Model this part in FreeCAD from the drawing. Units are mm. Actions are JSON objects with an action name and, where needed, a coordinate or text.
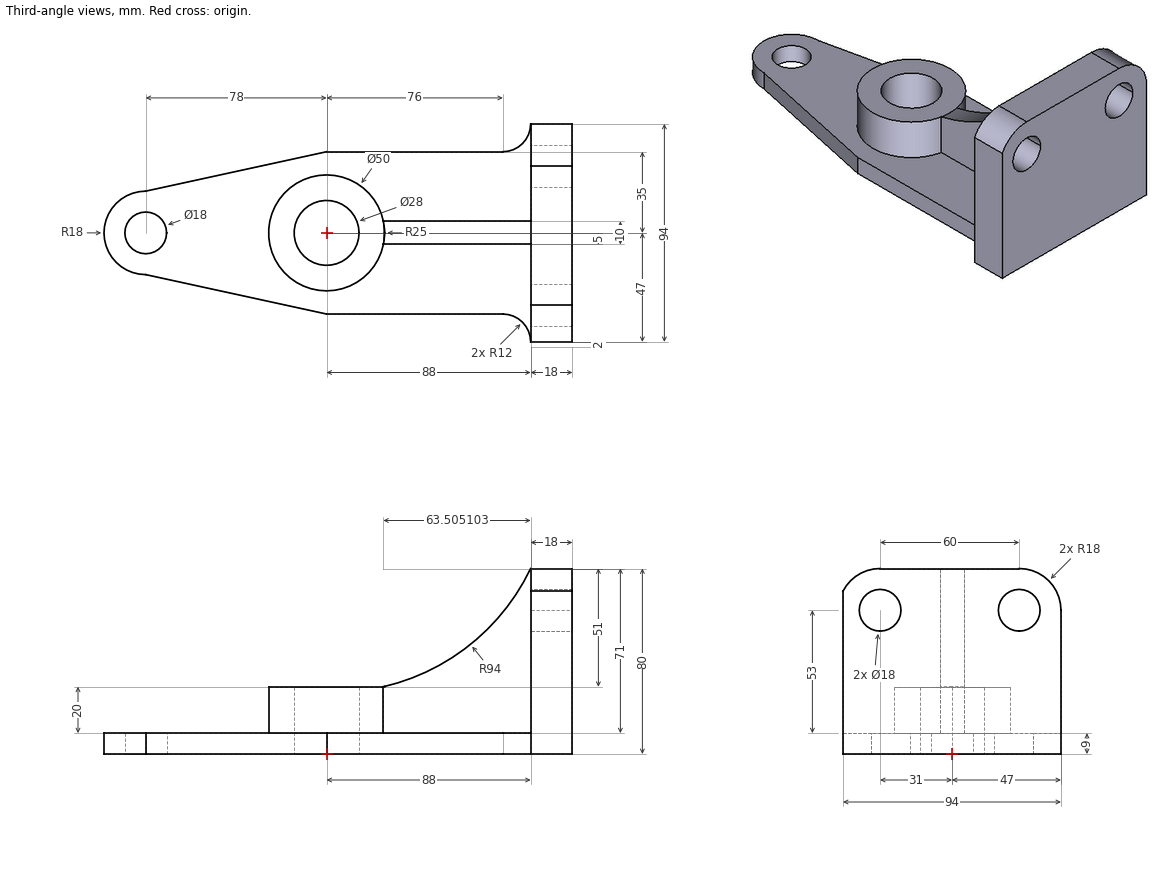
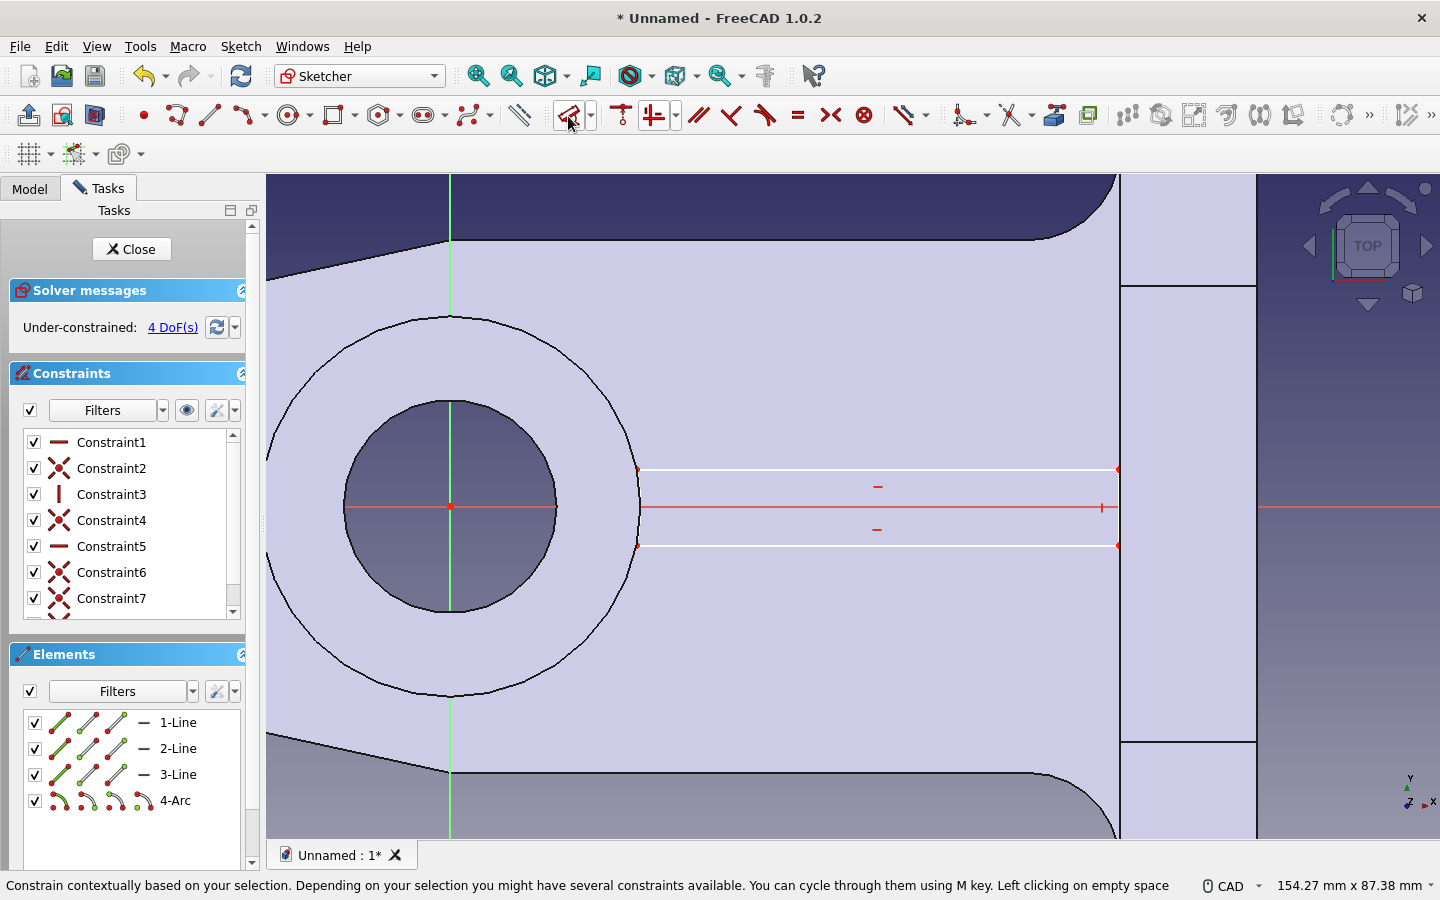
{"action": "left_click", "coordinate": [640, 523]}
{"action": "left_click", "coordinate": [672, 526]}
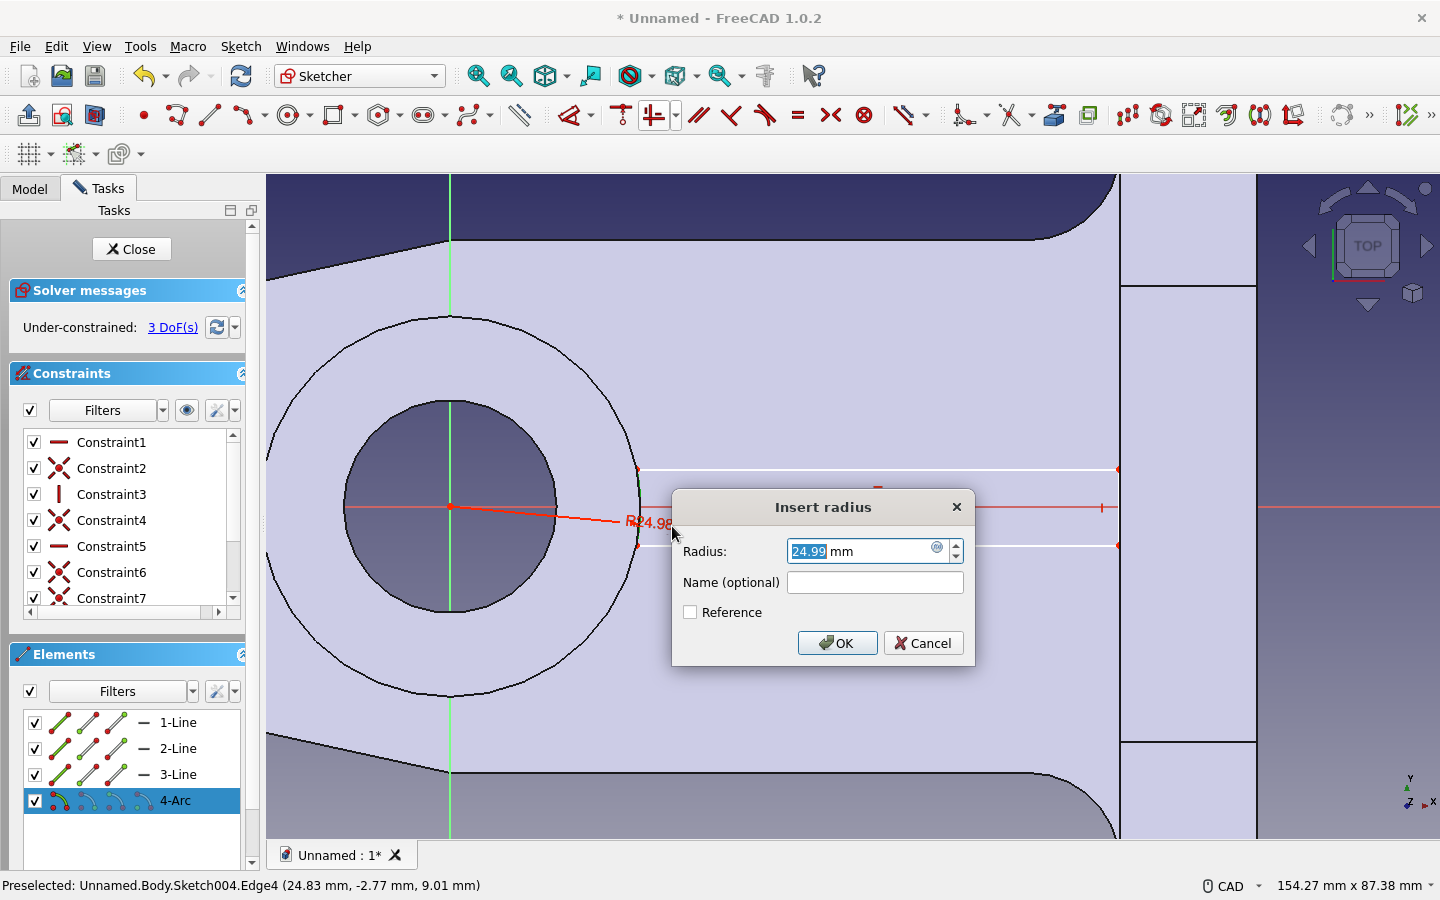
{"action": "type", "text": "25"}
{"action": "key", "text": "Return"}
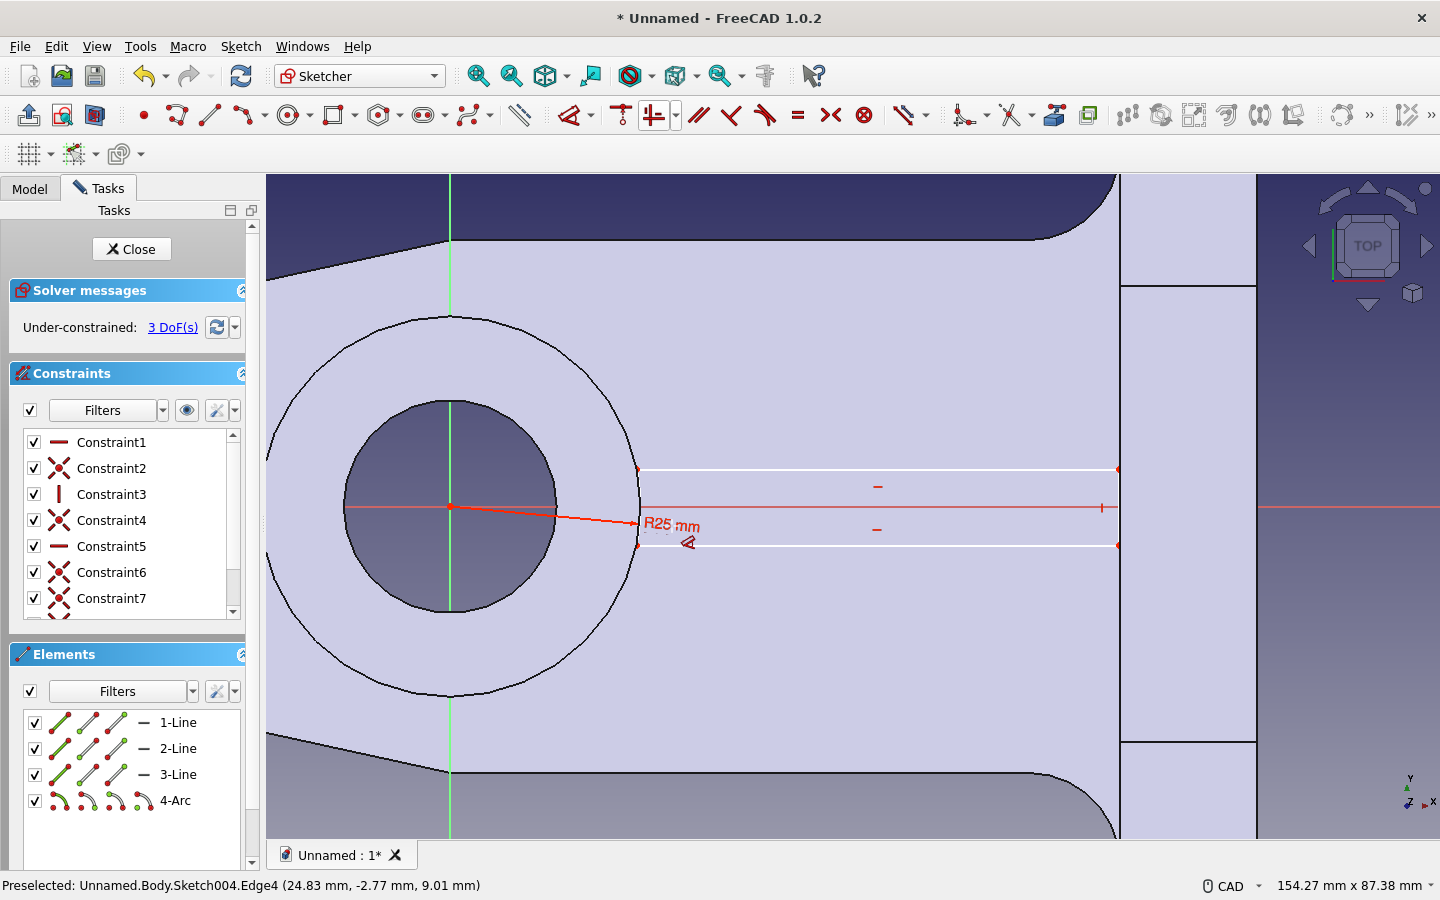
{"action": "left_click", "coordinate": [1119, 523]}
{"action": "left_click", "coordinate": [1153, 490]}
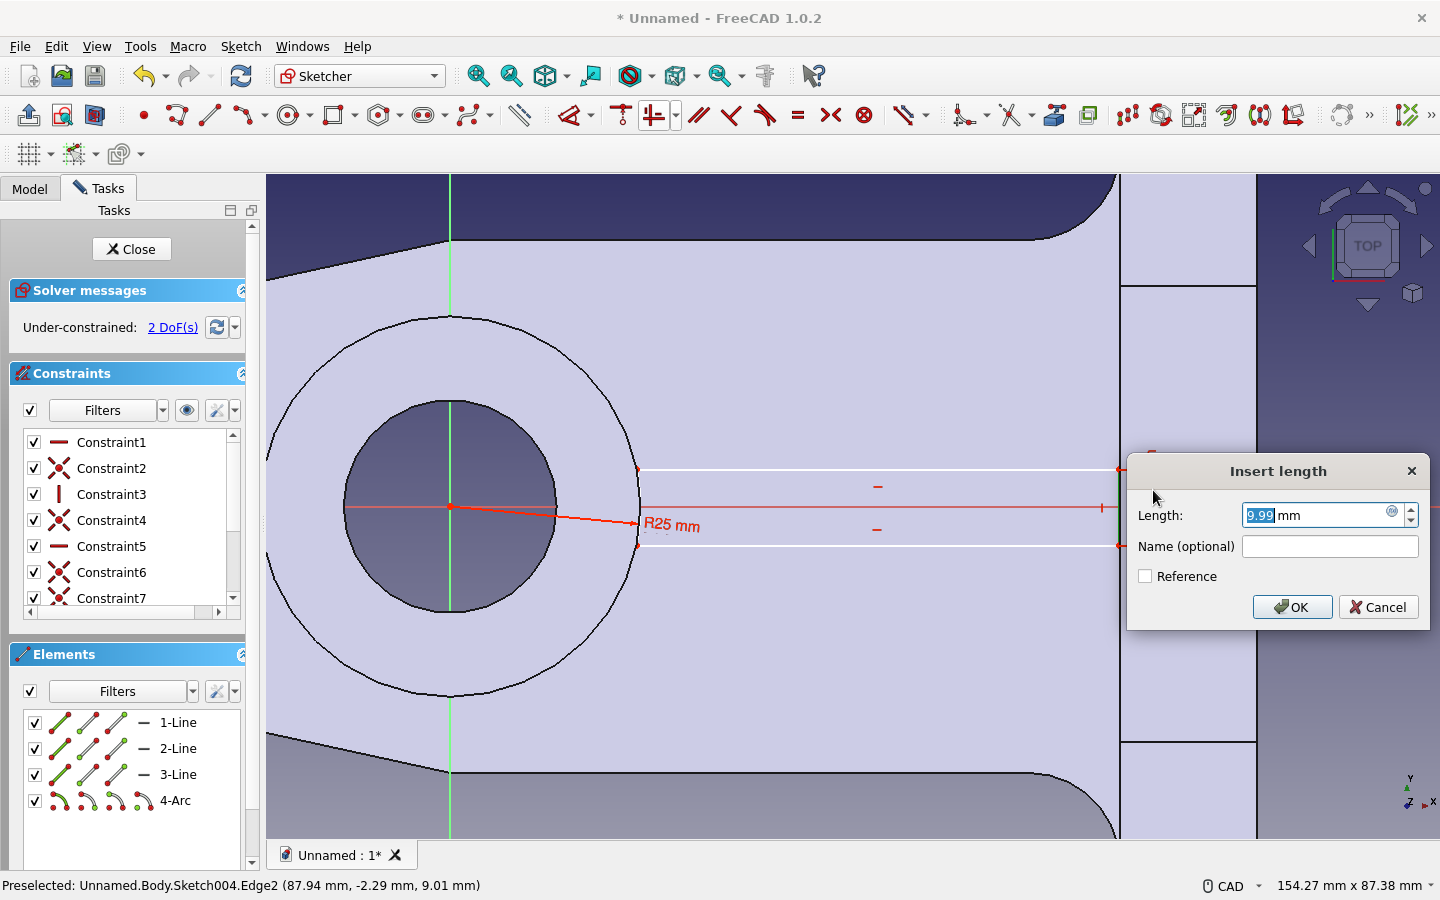
{"action": "type", "text": "10"}
{"action": "key", "text": "Return"}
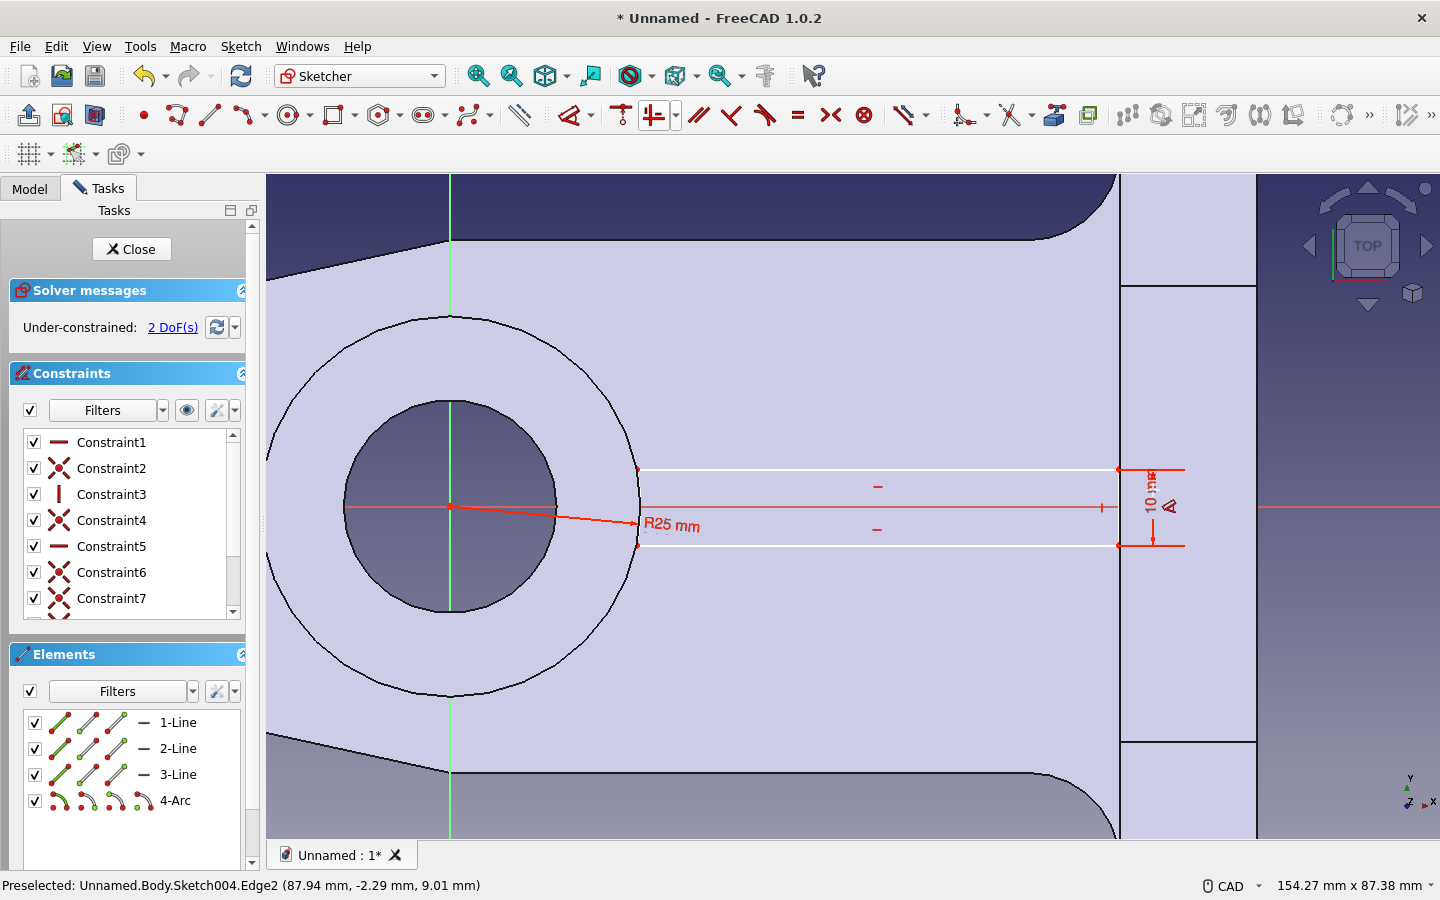
{"action": "left_click", "coordinate": [636, 546]}
{"action": "left_click", "coordinate": [416, 526]}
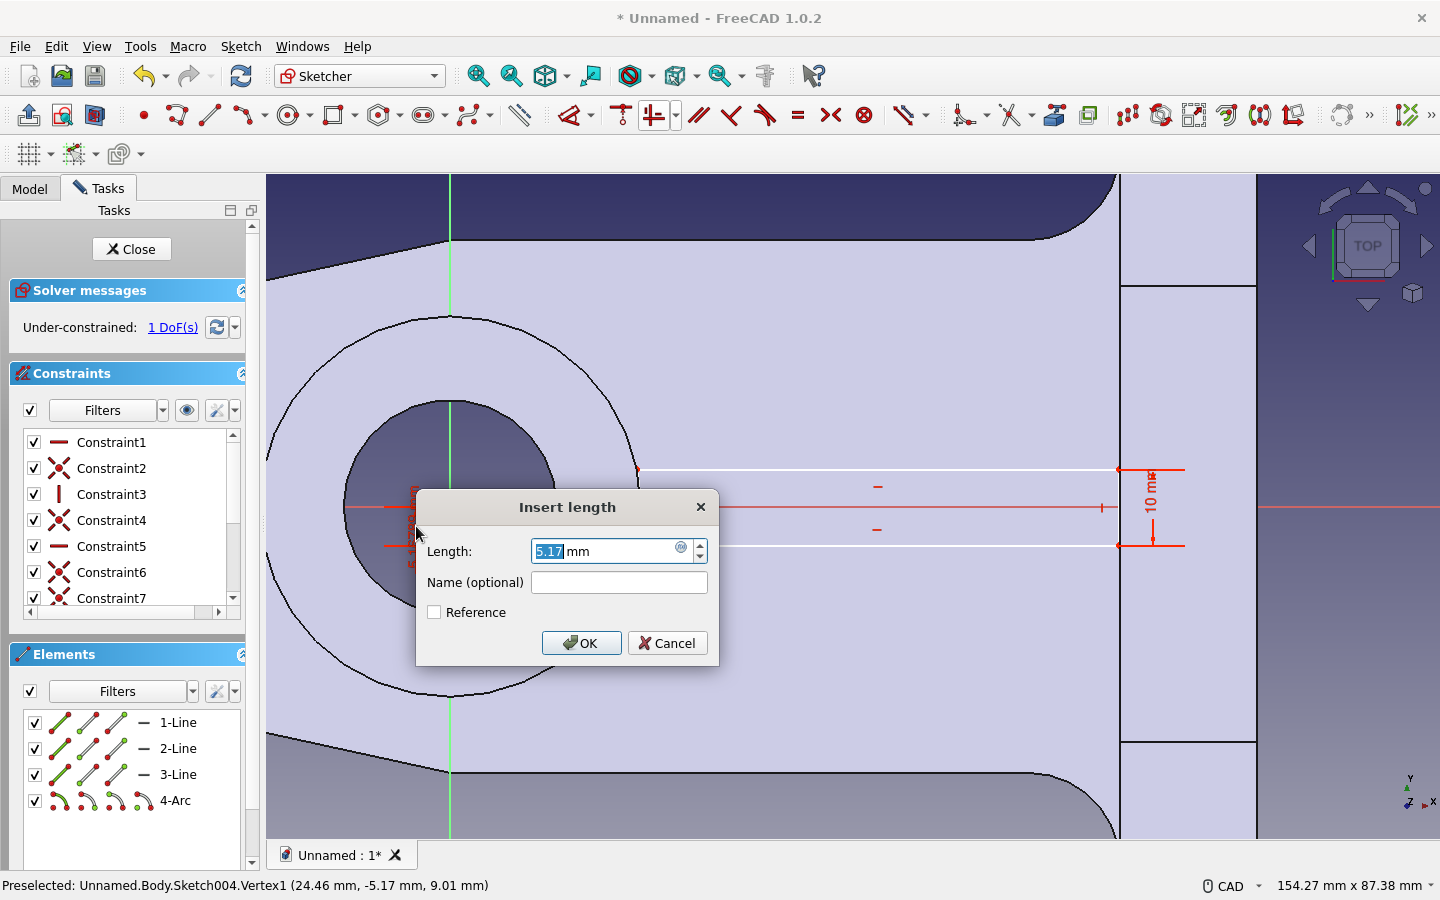
{"action": "type", "text": "5"}
{"action": "key", "text": "Return"}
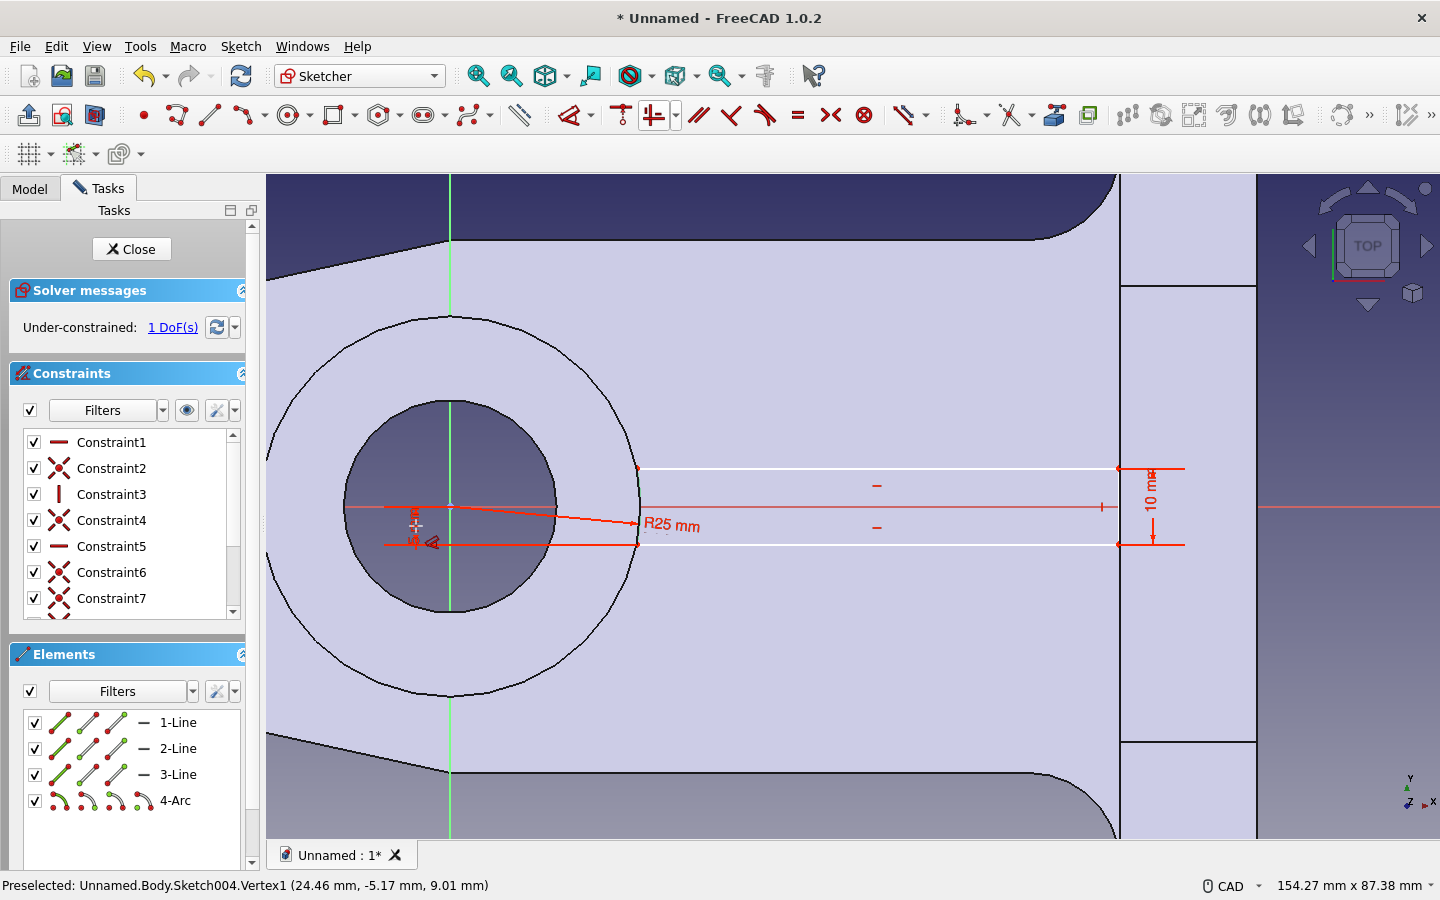
{"action": "left_click", "coordinate": [1119, 545]}
{"action": "left_click", "coordinate": [785, 579]}